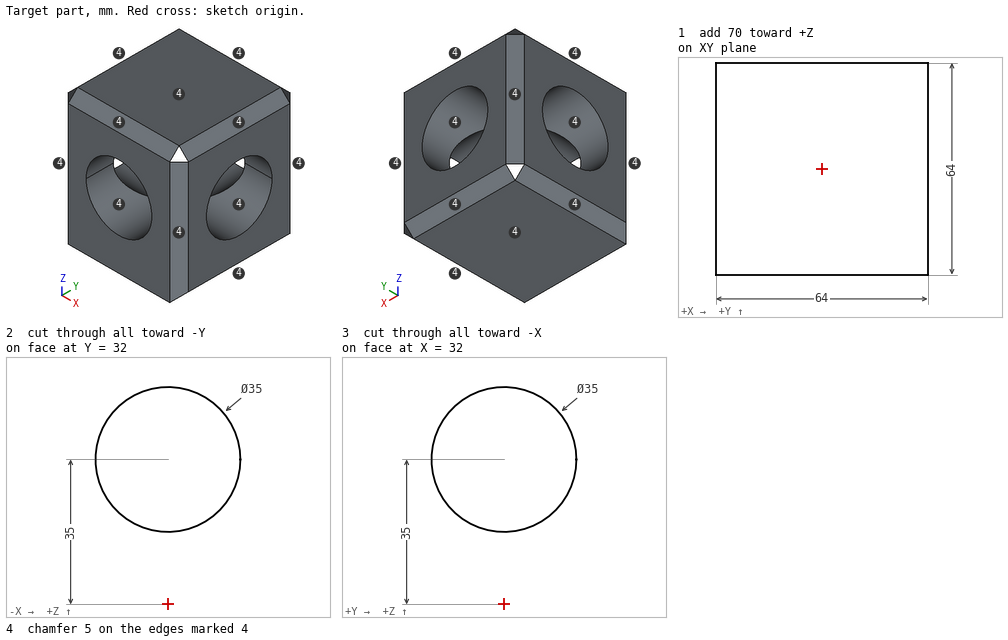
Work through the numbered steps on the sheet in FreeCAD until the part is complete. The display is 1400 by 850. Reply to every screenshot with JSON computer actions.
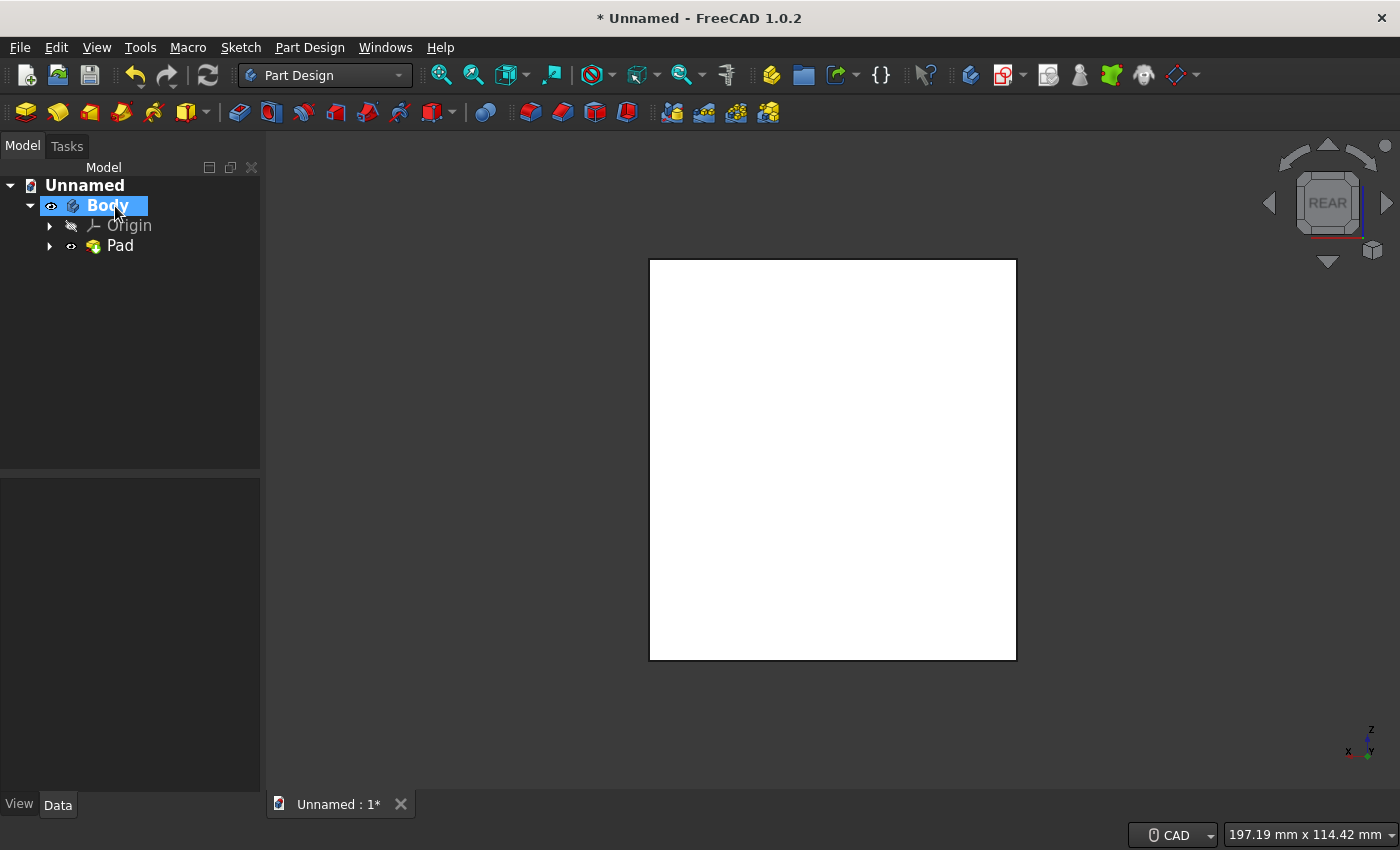
{"action": "left_click", "coordinate": [833, 459]}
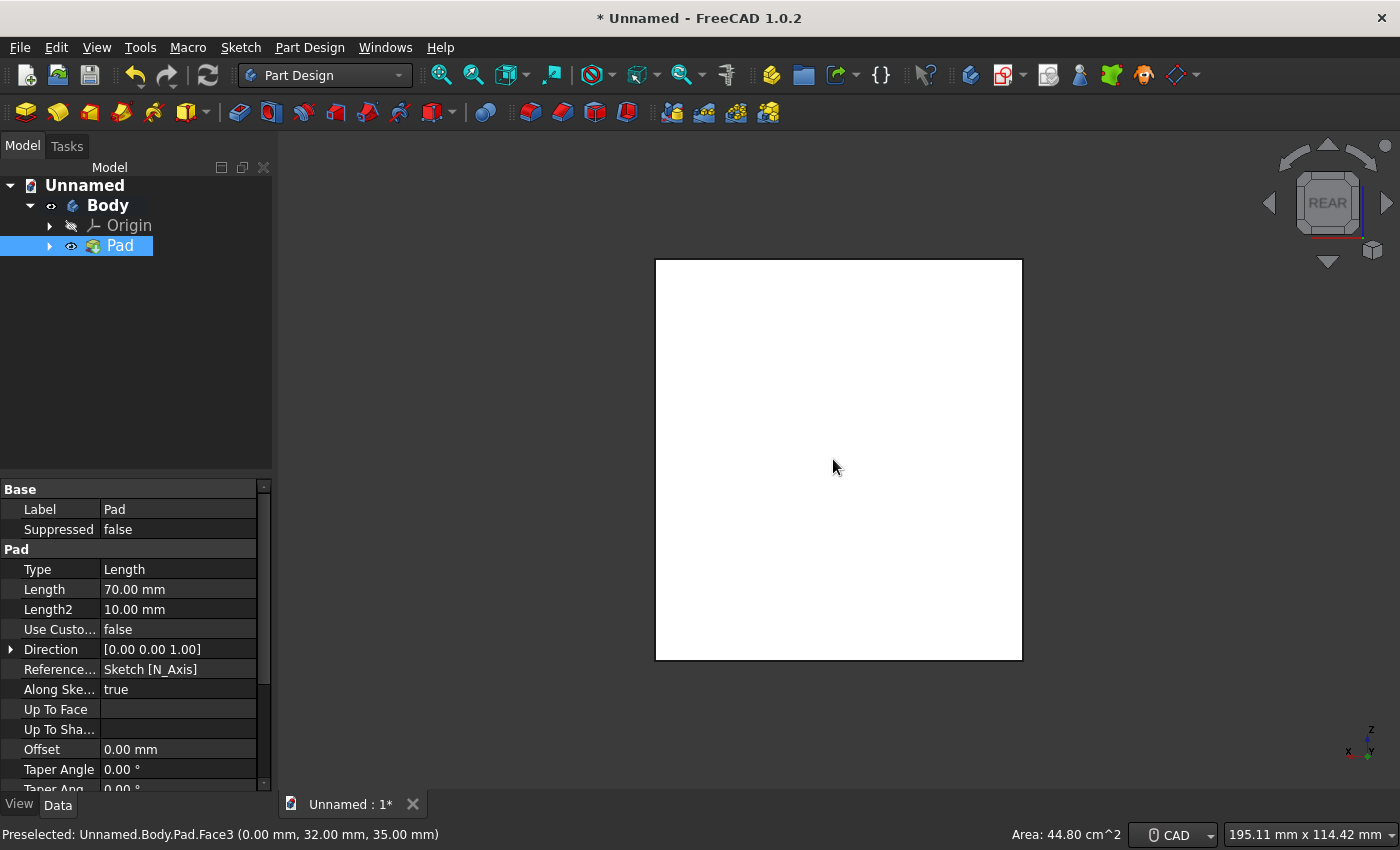
{"action": "left_click", "coordinate": [1004, 76]}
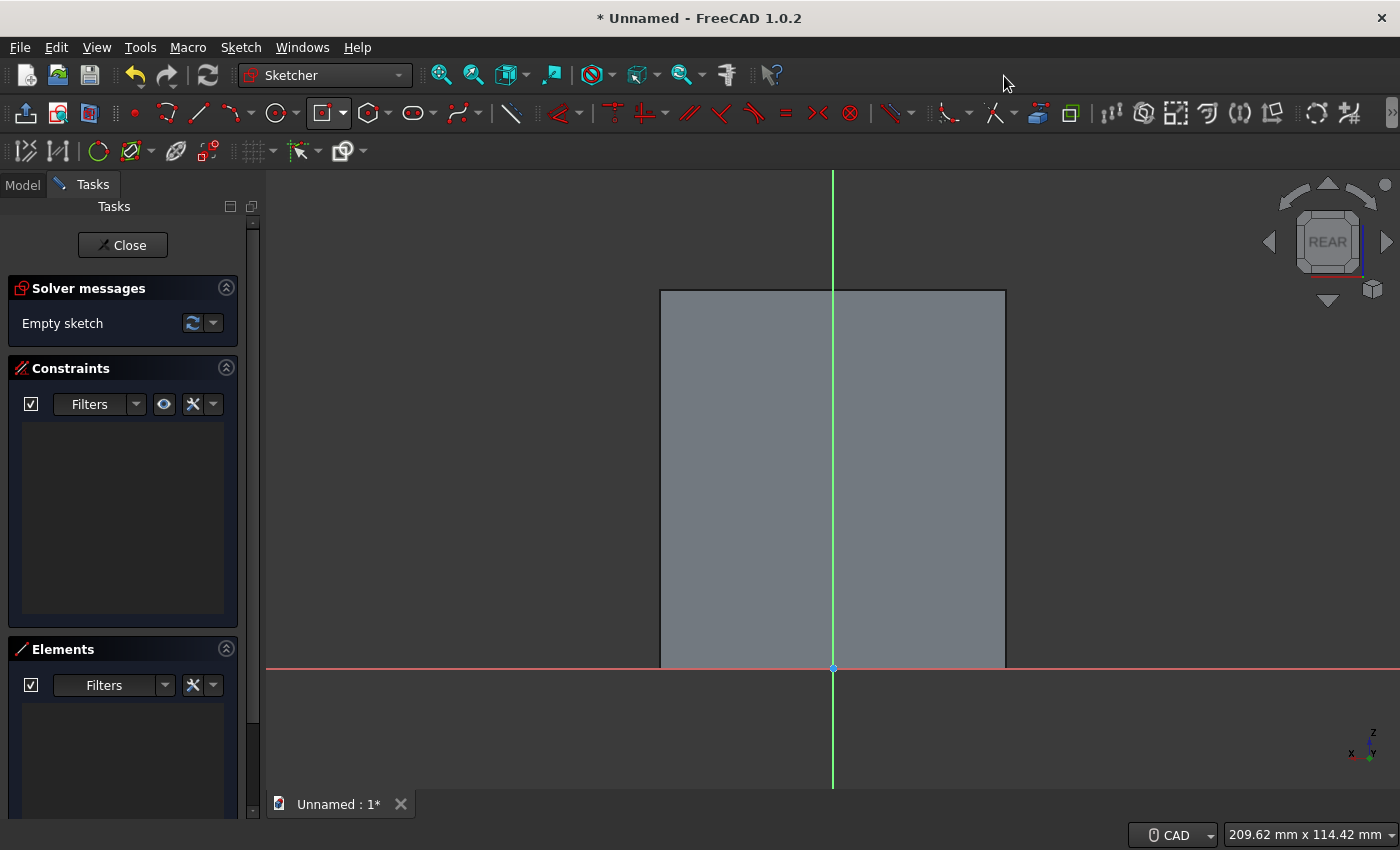
{"action": "scroll", "coordinate": [972, 623], "scroll_direction": "up", "scroll_amount": 2}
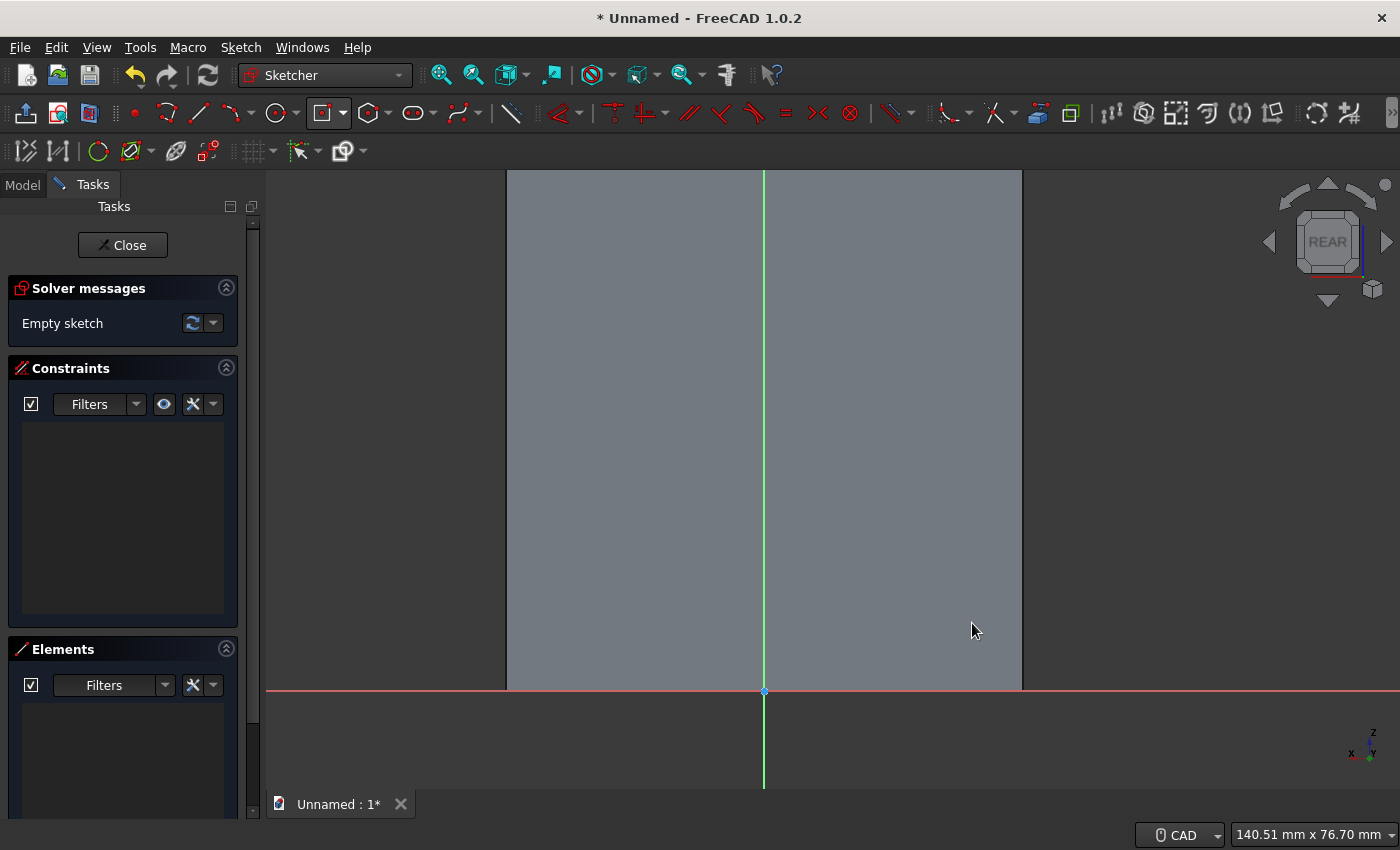
{"action": "key", "text": "g c"}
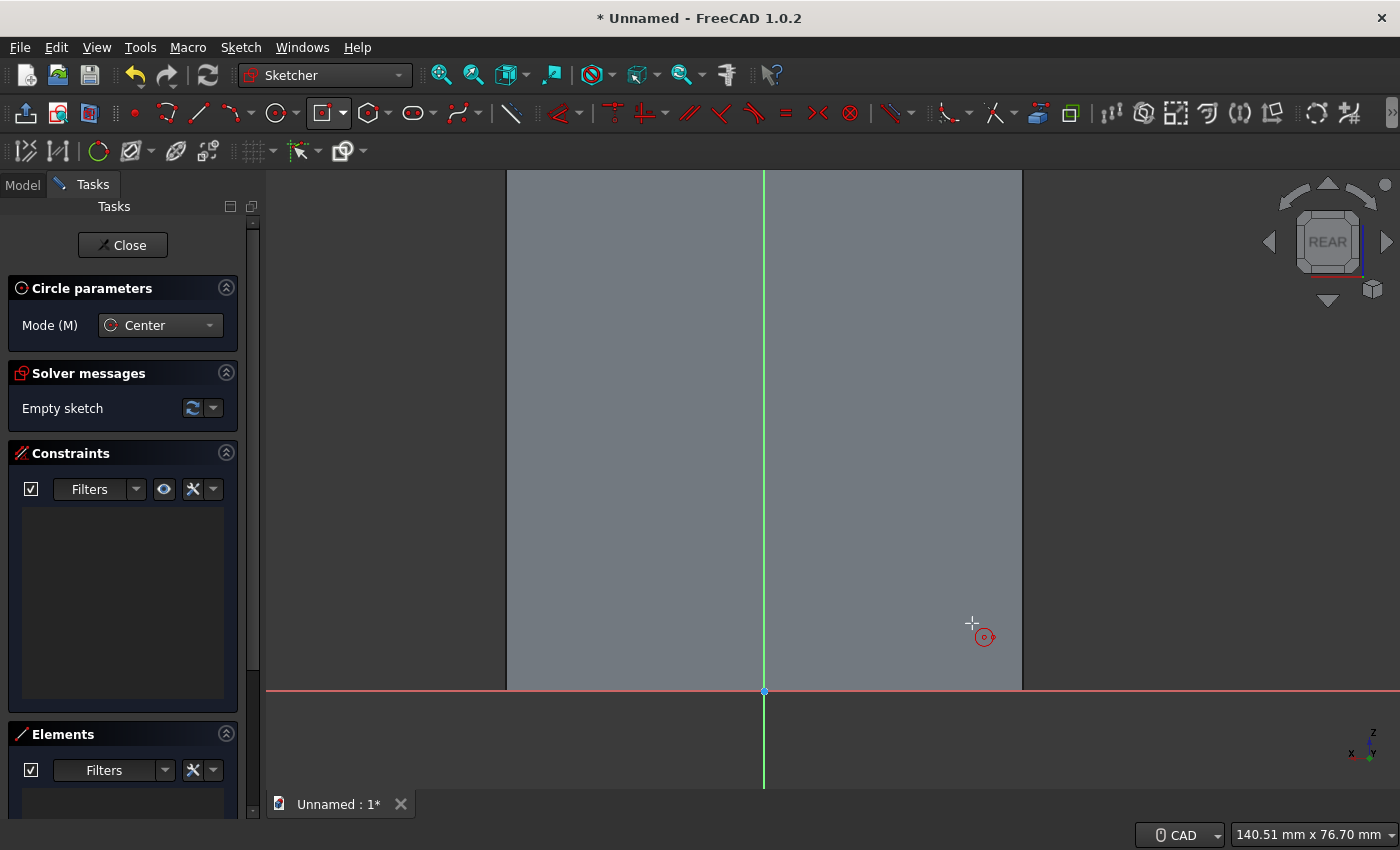
{"action": "left_click", "coordinate": [764, 409]}
{"action": "left_click", "coordinate": [864, 309]}
{"action": "key", "text": "Escape"}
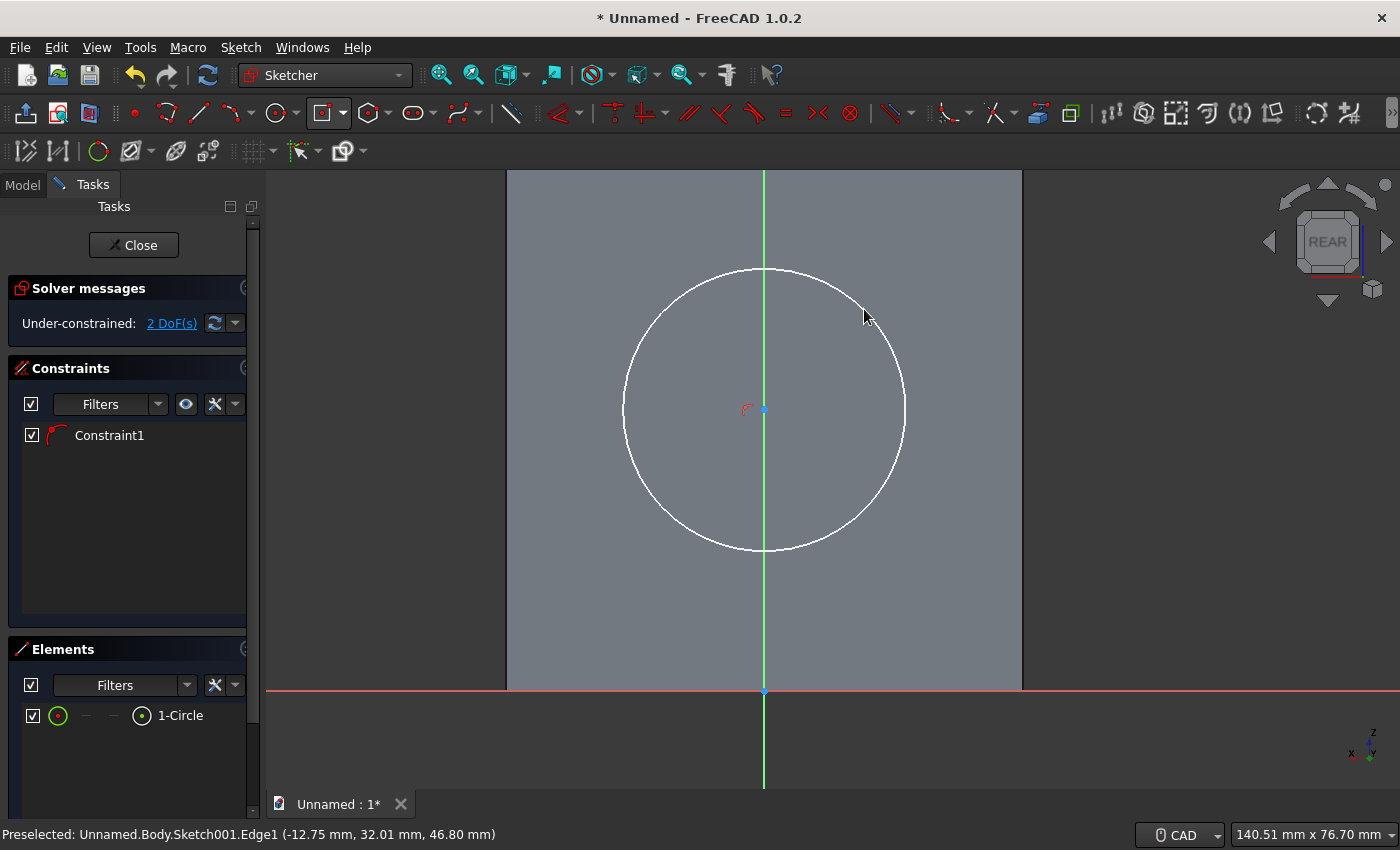
{"action": "left_click", "coordinate": [558, 114]}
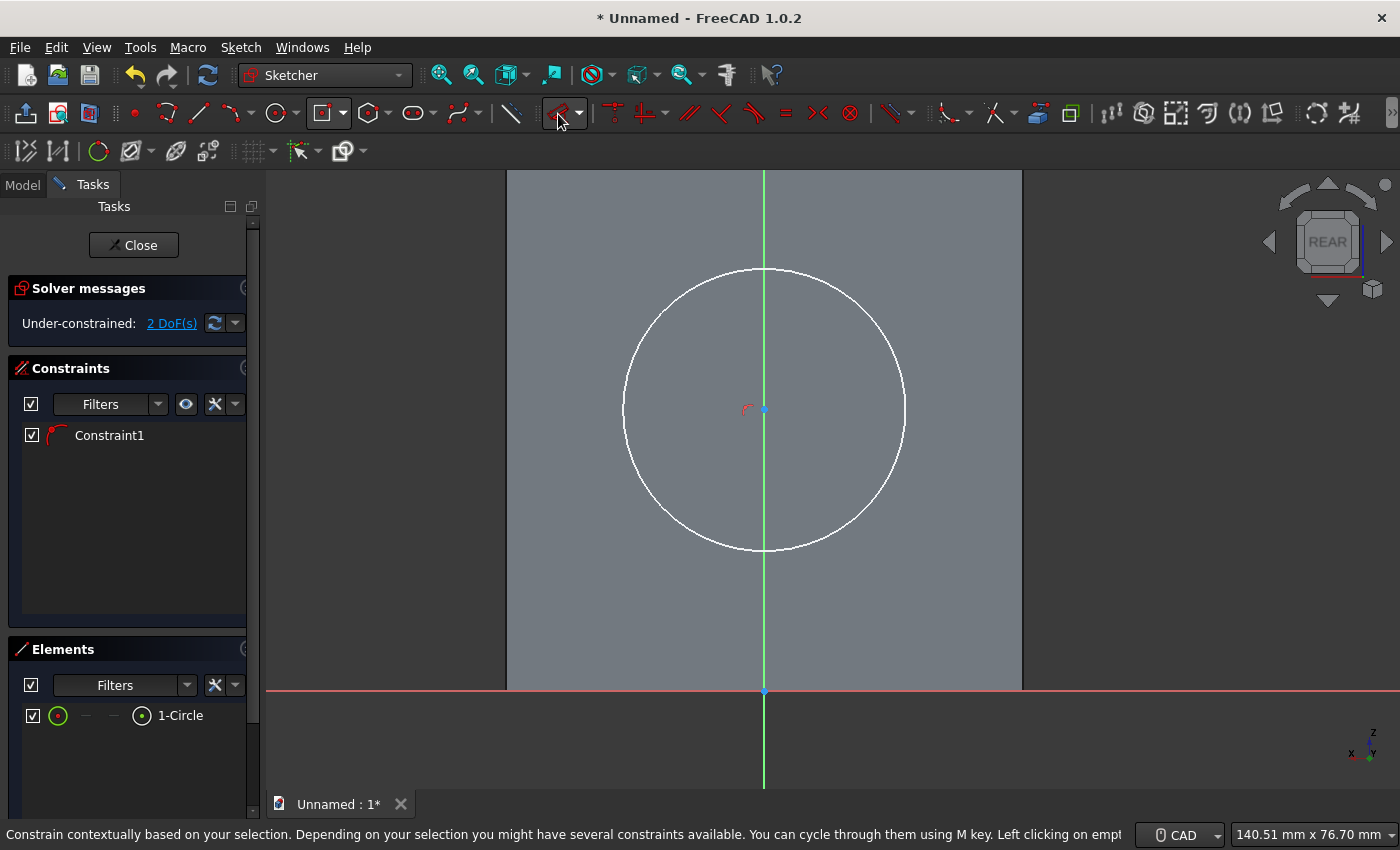
{"action": "left_click", "coordinate": [864, 310]}
{"action": "left_click", "coordinate": [887, 287]}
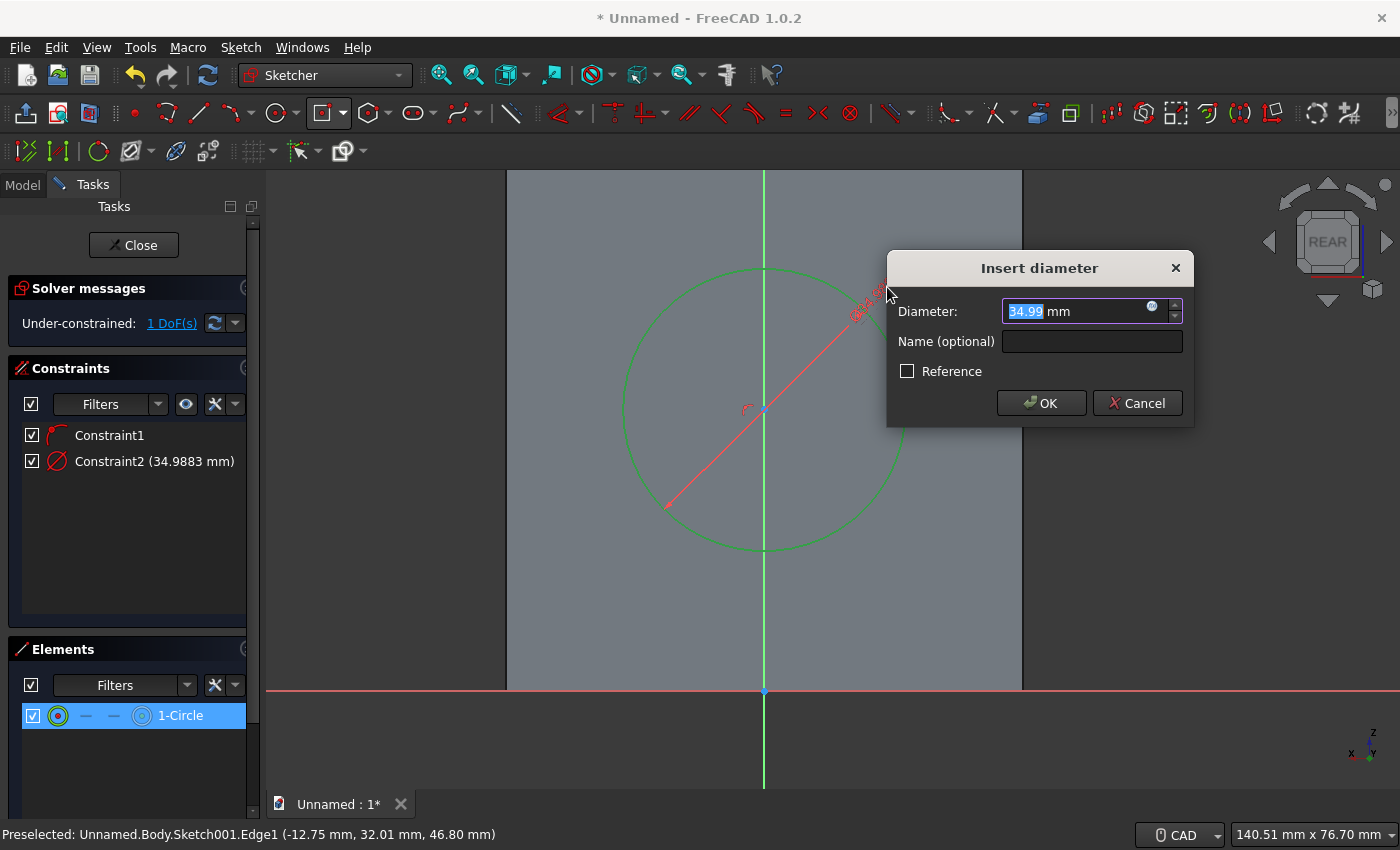
{"action": "type", "text": "35"}
{"action": "key", "text": "Return"}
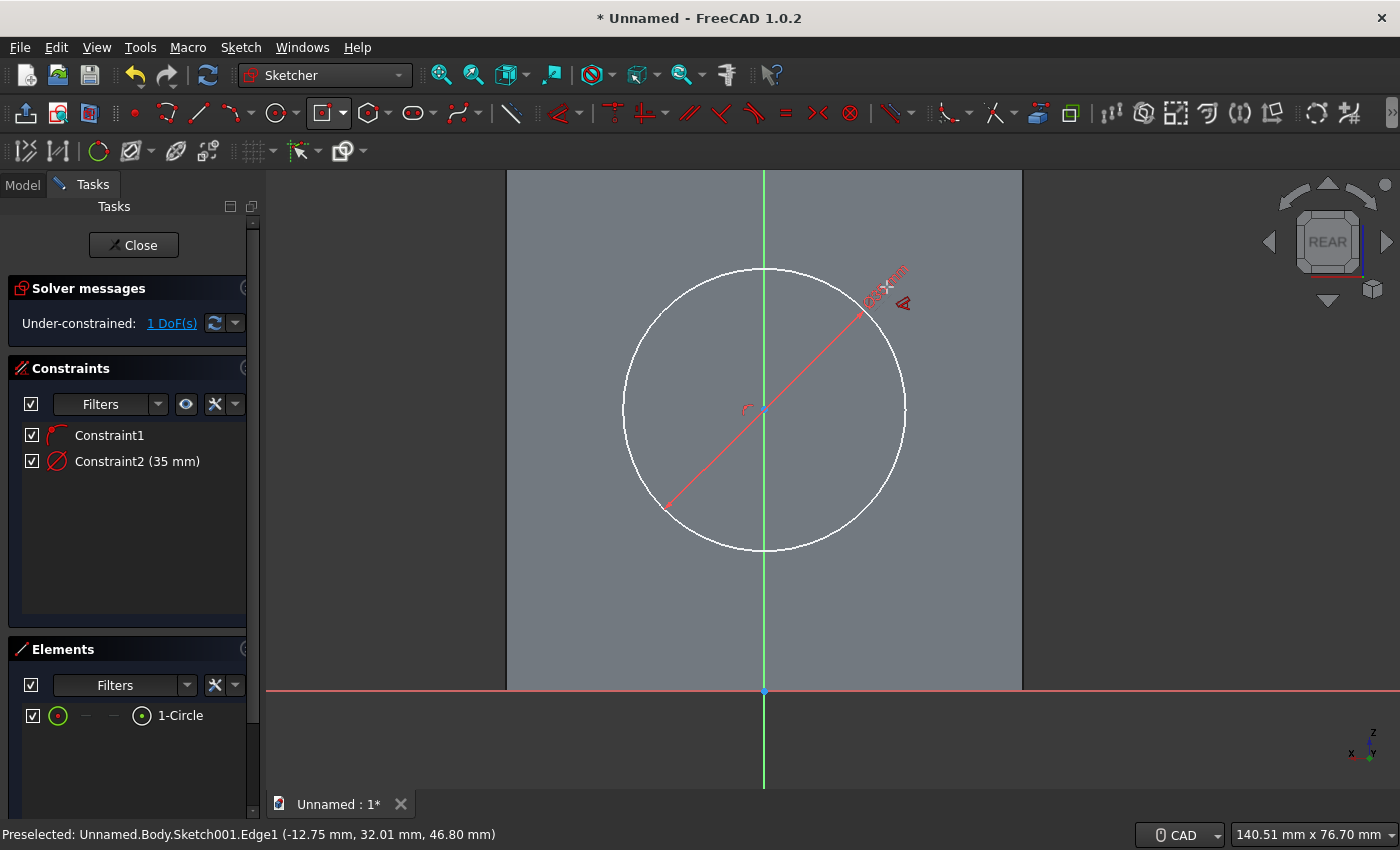
{"action": "left_click", "coordinate": [764, 410]}
{"action": "left_click", "coordinate": [798, 486]}